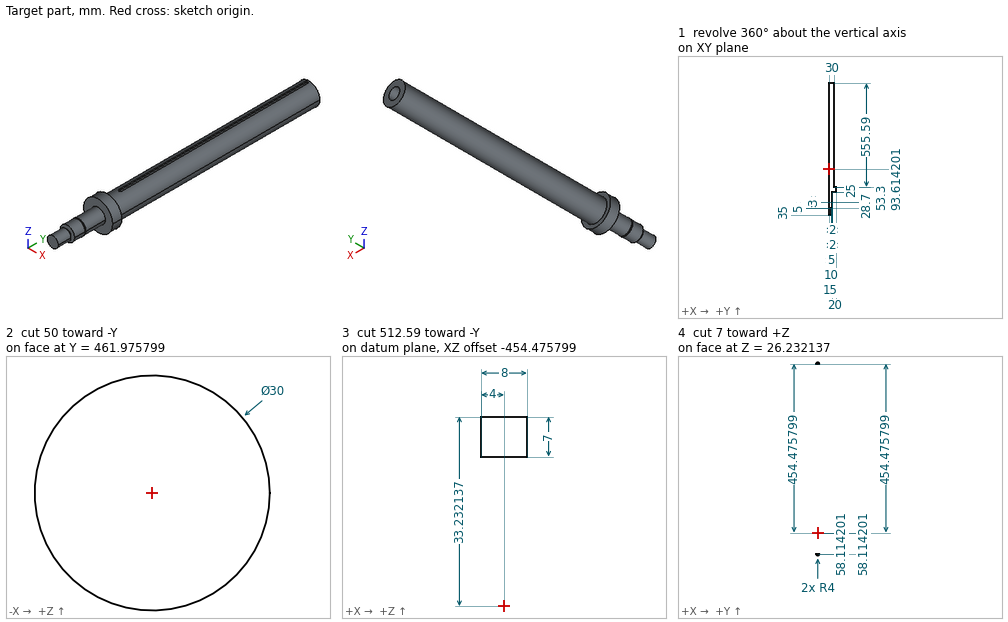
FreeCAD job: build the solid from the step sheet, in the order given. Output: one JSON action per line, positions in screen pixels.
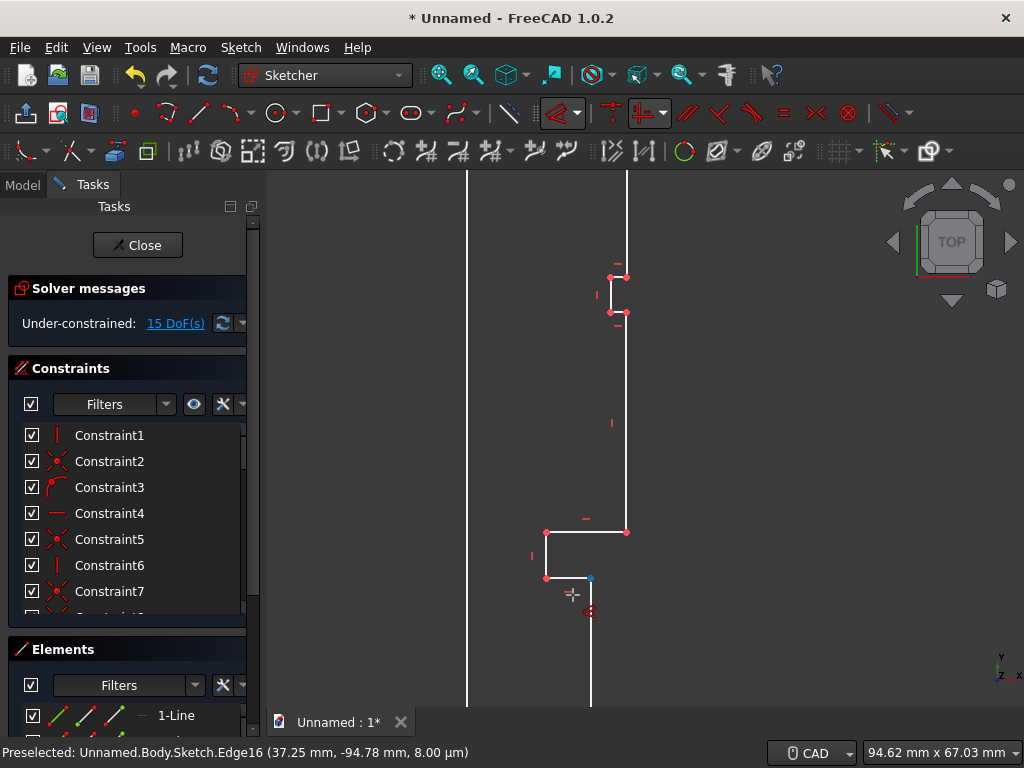
{"action": "left_click", "coordinate": [573, 578]}
{"action": "left_click", "coordinate": [568, 612]}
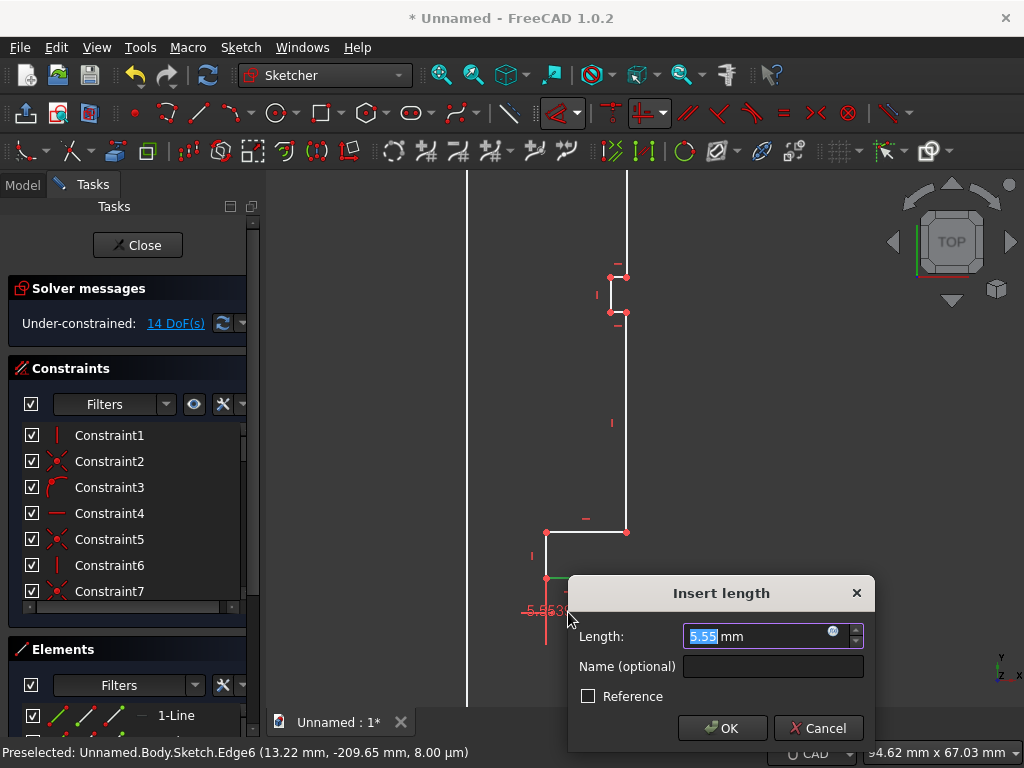
{"action": "type", "text": "5"}
{"action": "key", "text": "Return"}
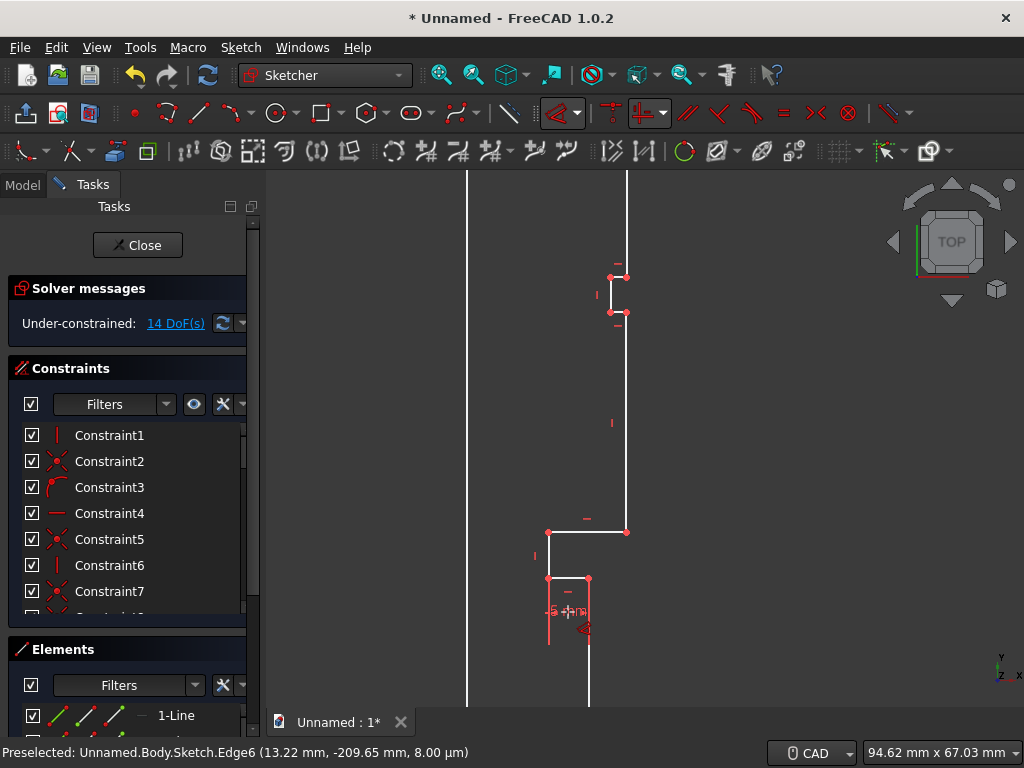
{"action": "left_click", "coordinate": [549, 564]}
{"action": "left_click", "coordinate": [515, 555]}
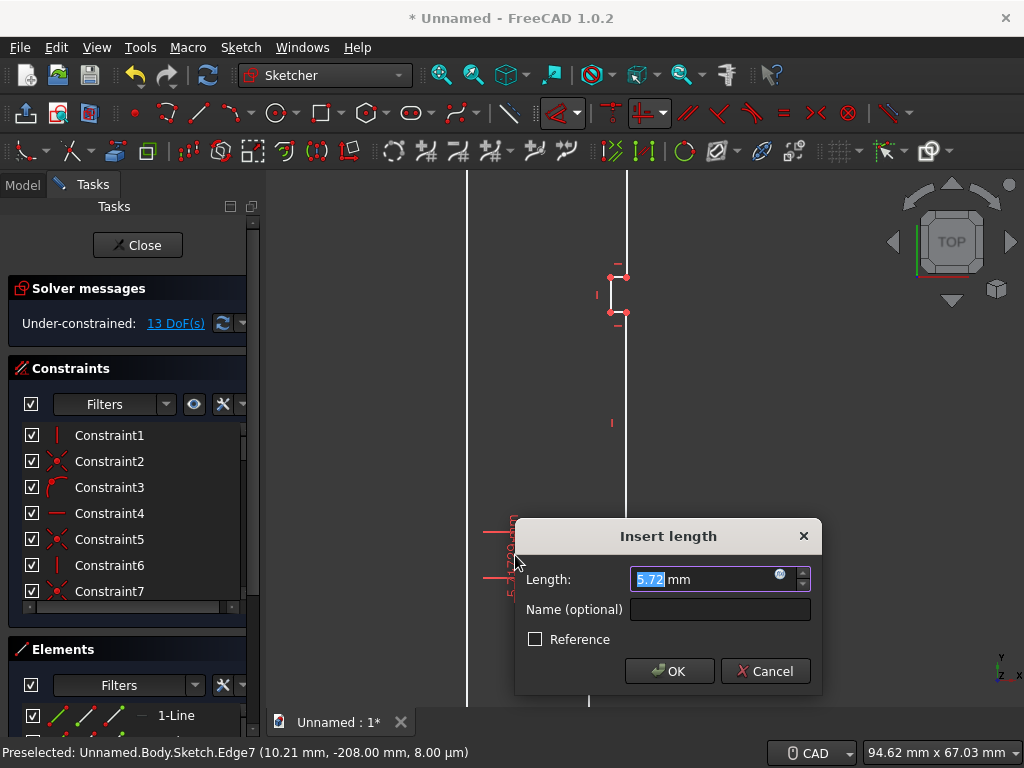
{"action": "type", "text": "5"}
{"action": "key", "text": "Return"}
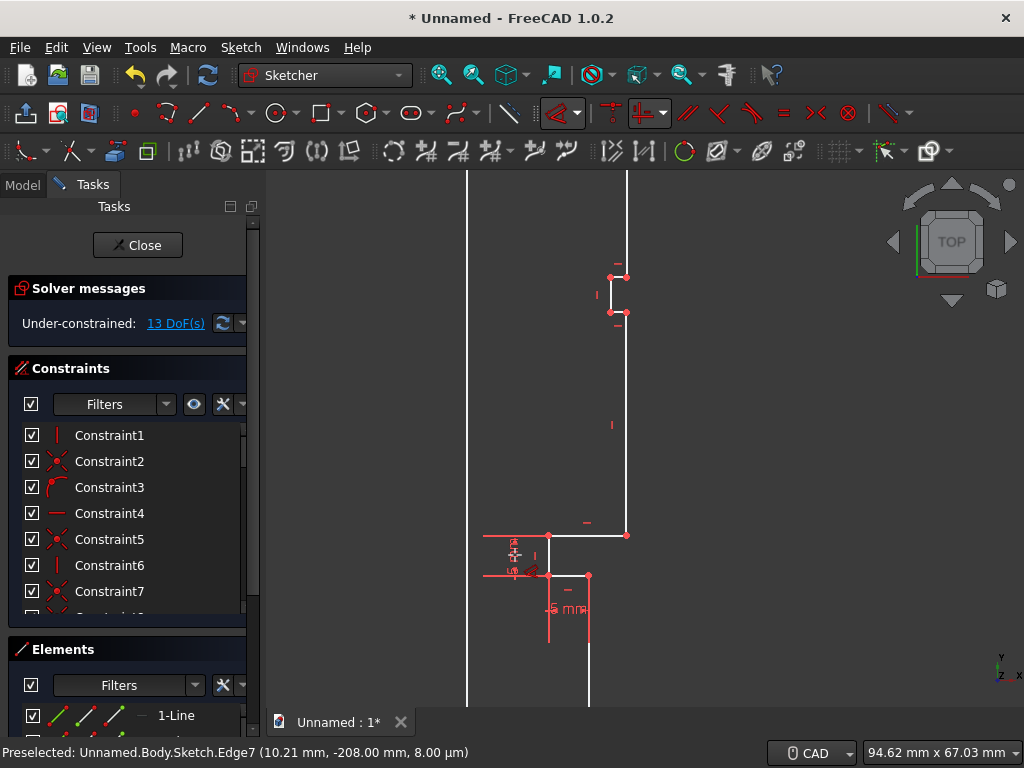
{"action": "scroll", "coordinate": [619, 312], "scroll_direction": "up", "scroll_amount": 5}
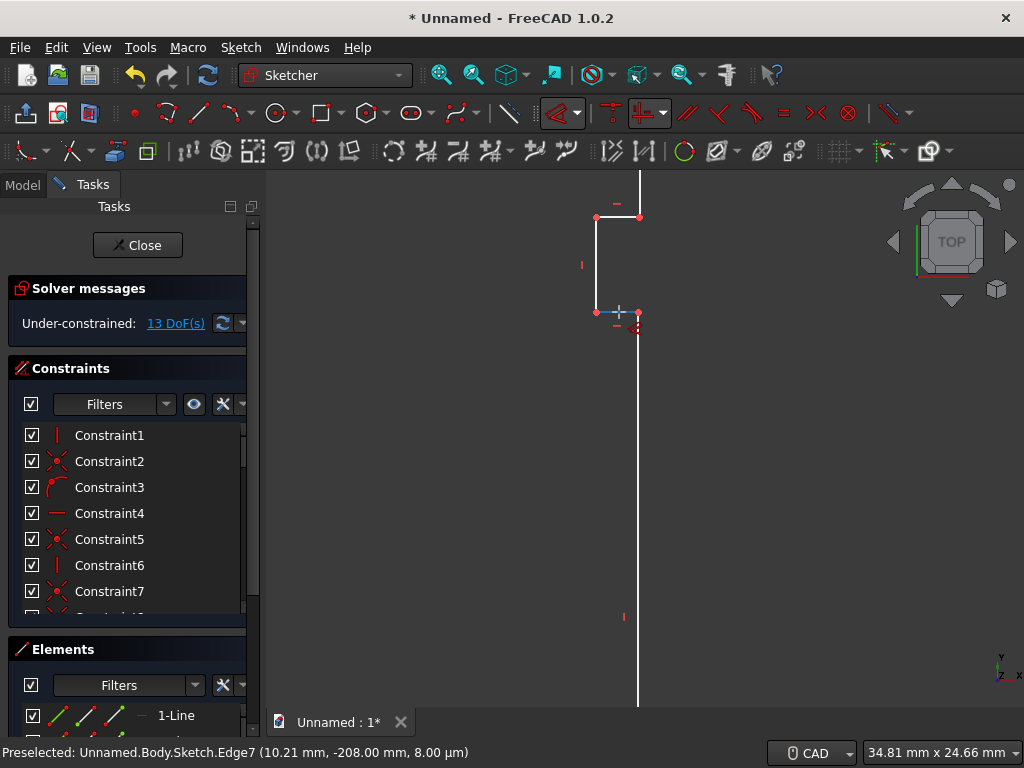
{"action": "left_click", "coordinate": [617, 312]}
{"action": "left_click", "coordinate": [617, 346]}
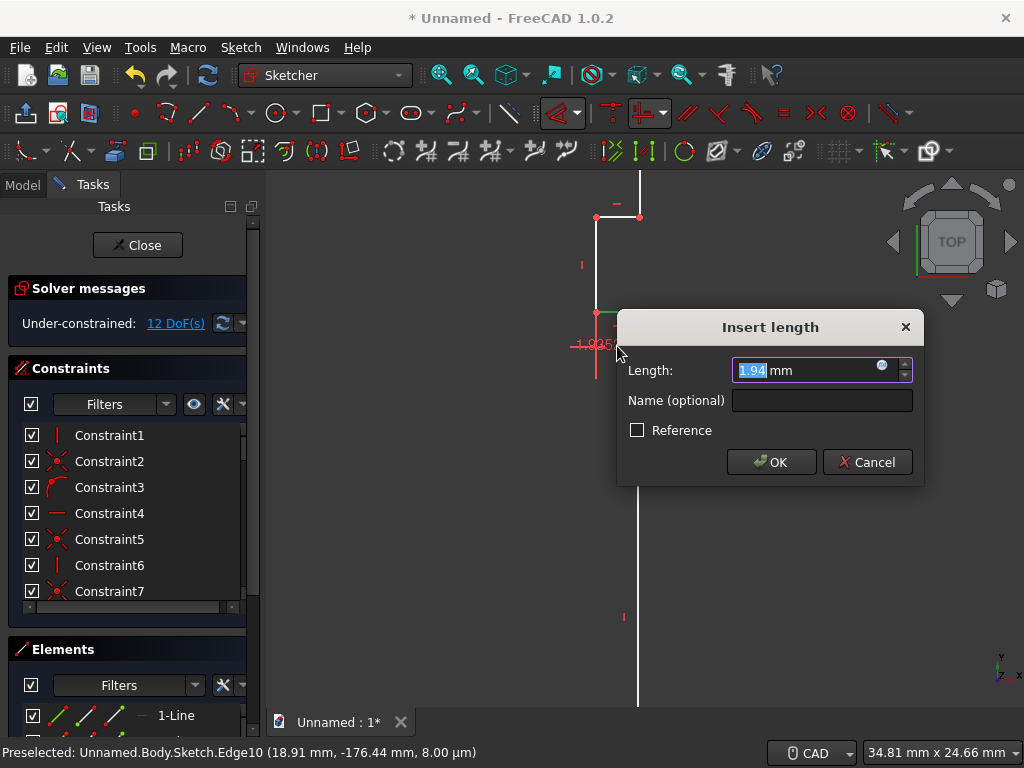
{"action": "type", "text": "2"}
{"action": "key", "text": "Return"}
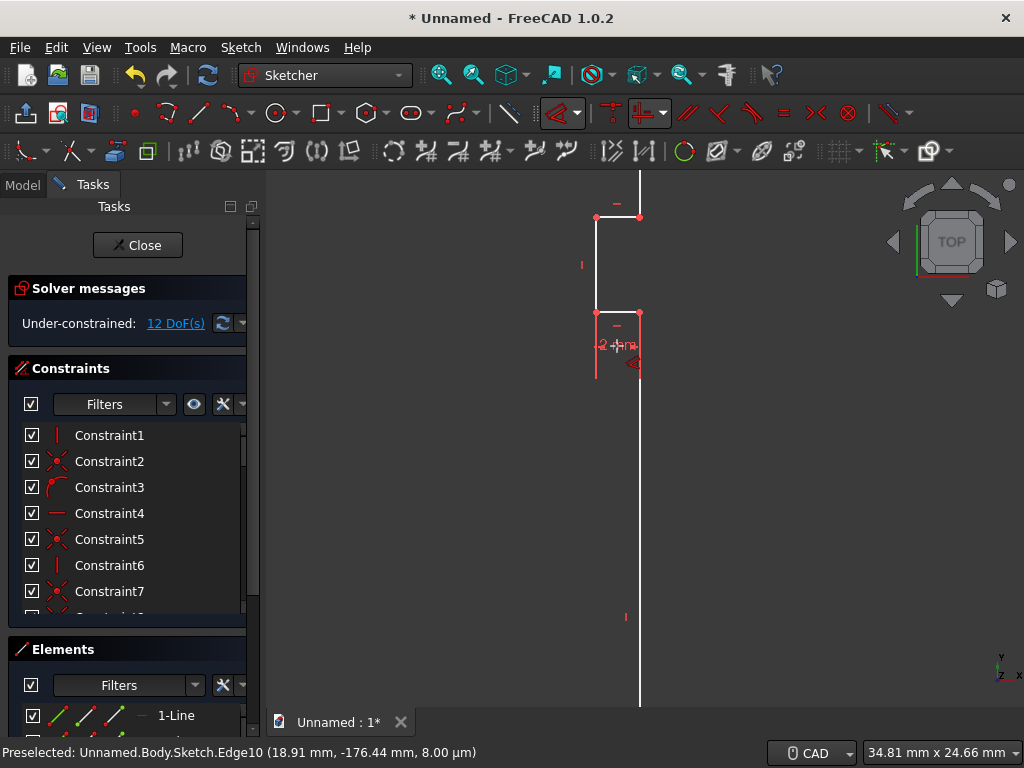
{"action": "left_click", "coordinate": [596, 284]}
{"action": "left_click", "coordinate": [562, 265]}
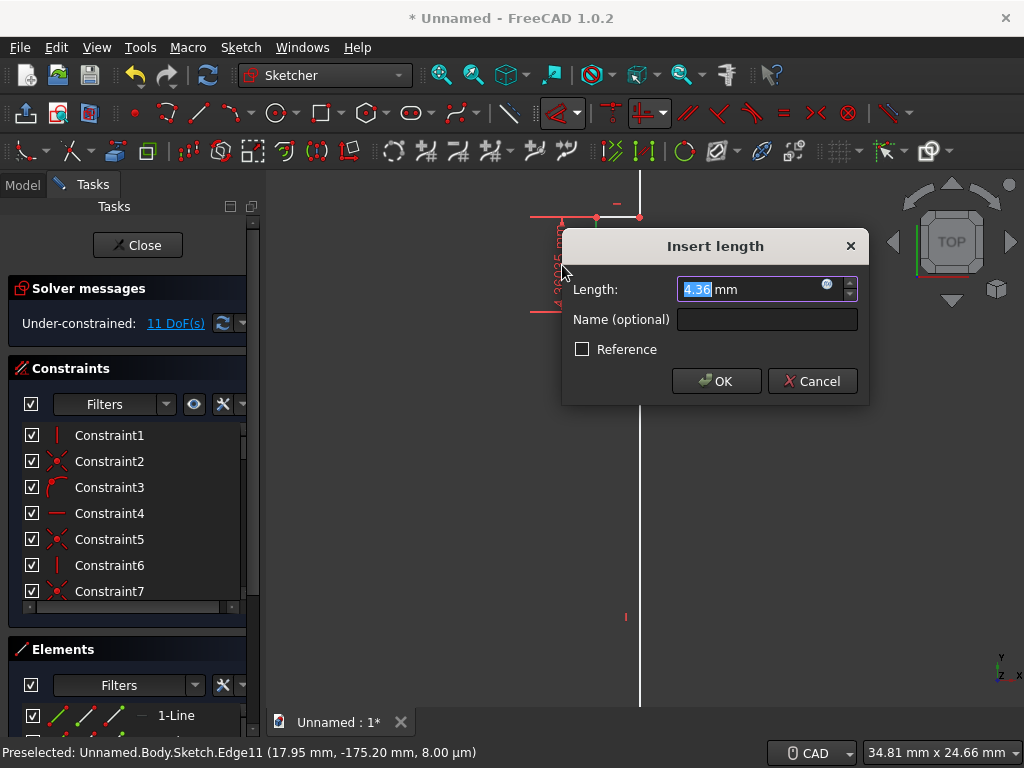
{"action": "type", "text": "3"}
{"action": "key", "text": "Return"}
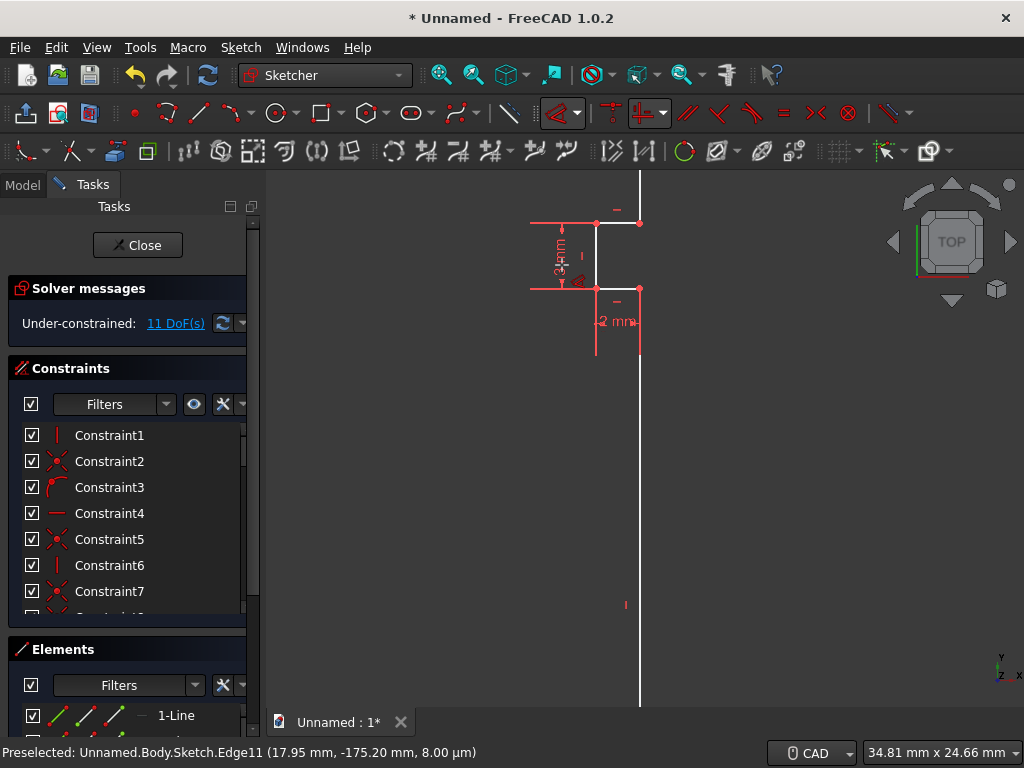
{"action": "left_click", "coordinate": [609, 223]}
{"action": "left_click", "coordinate": [633, 257]}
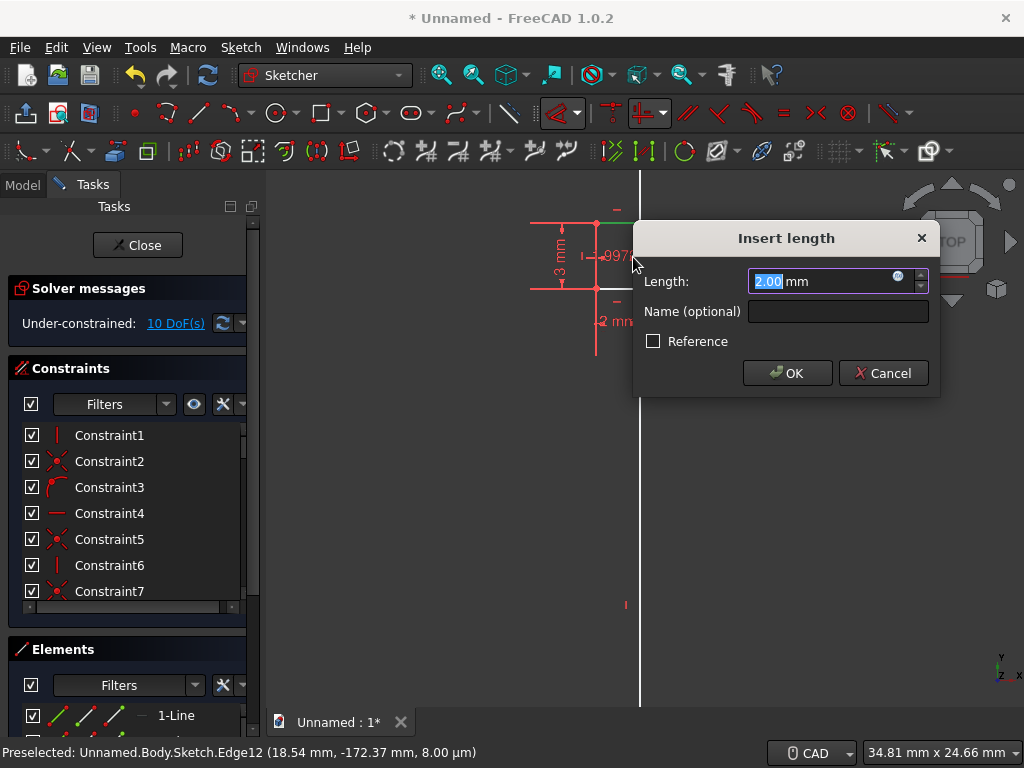
{"action": "type", "text": "2"}
{"action": "key", "text": "Return"}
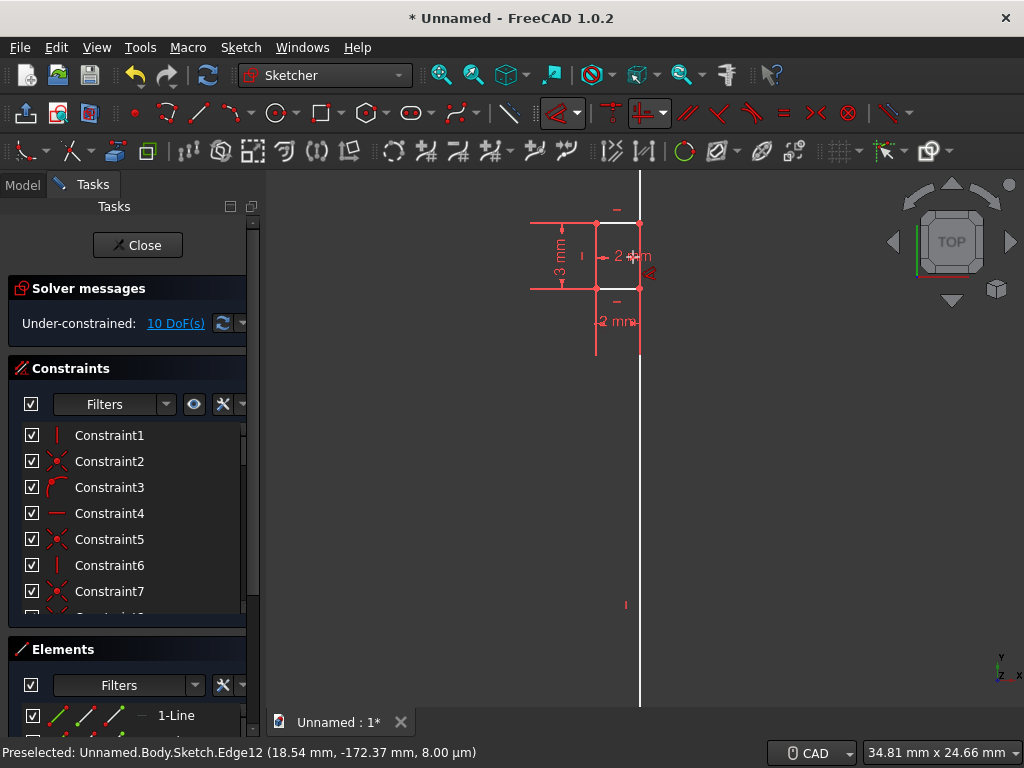
{"action": "scroll", "coordinate": [575, 617], "scroll_direction": "down", "scroll_amount": 18}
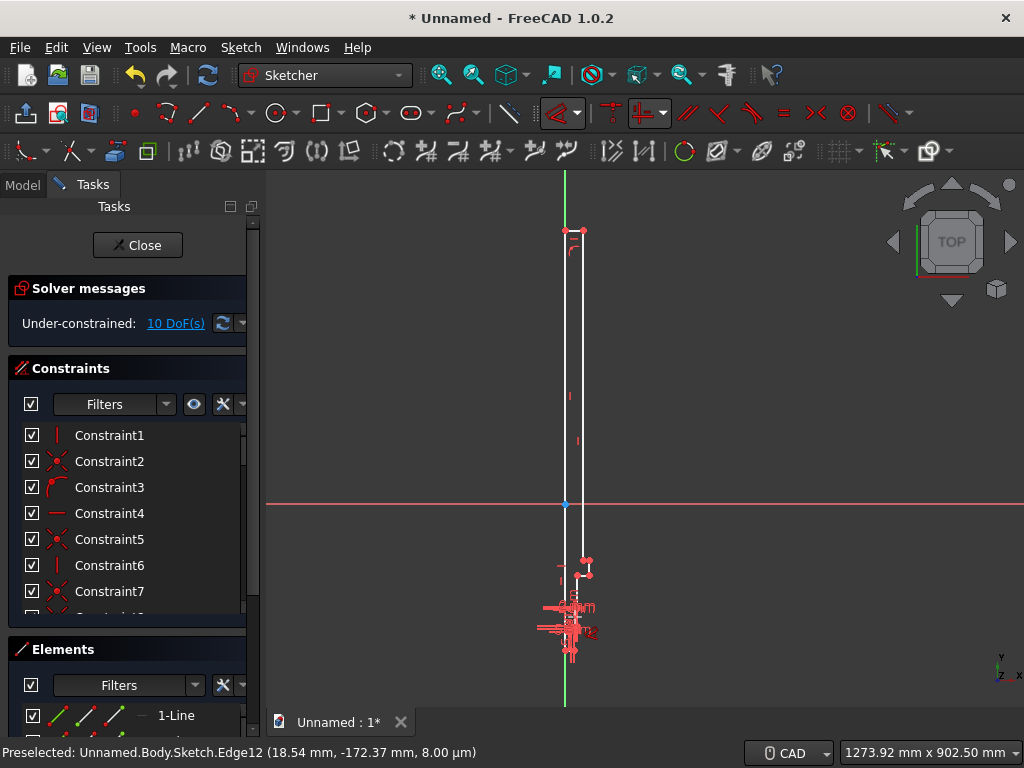
{"action": "scroll", "coordinate": [578, 231], "scroll_direction": "up", "scroll_amount": 5}